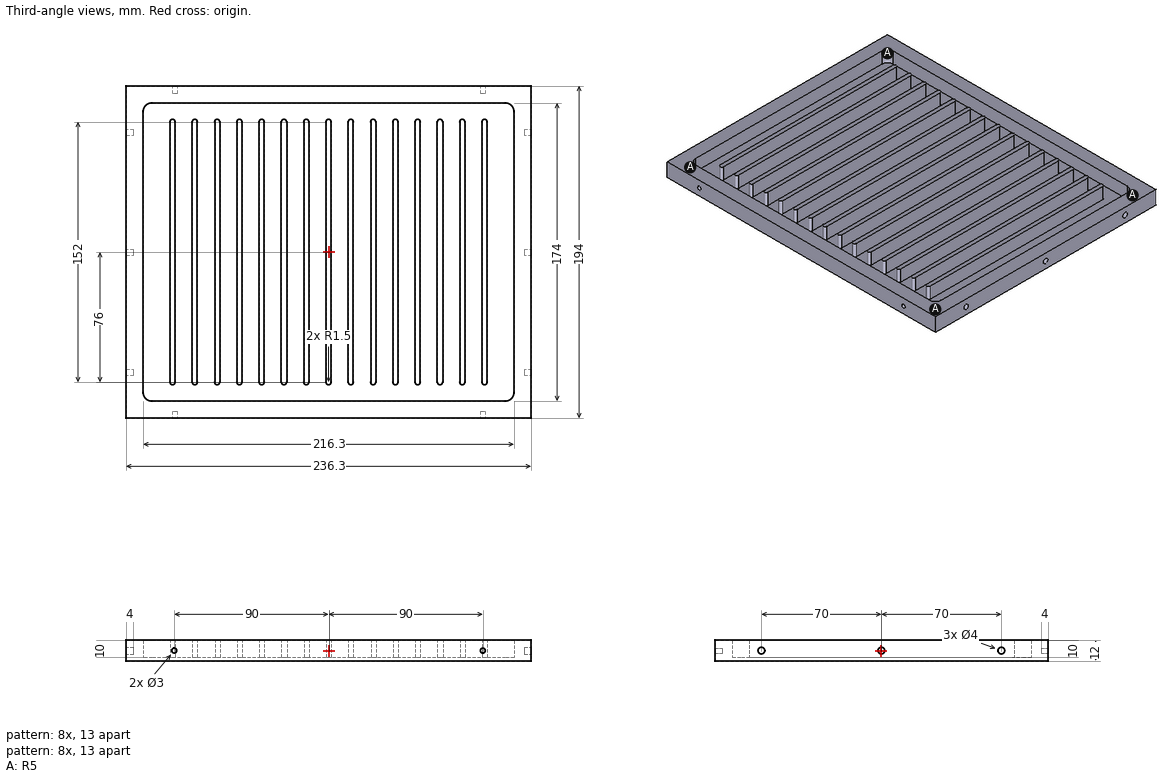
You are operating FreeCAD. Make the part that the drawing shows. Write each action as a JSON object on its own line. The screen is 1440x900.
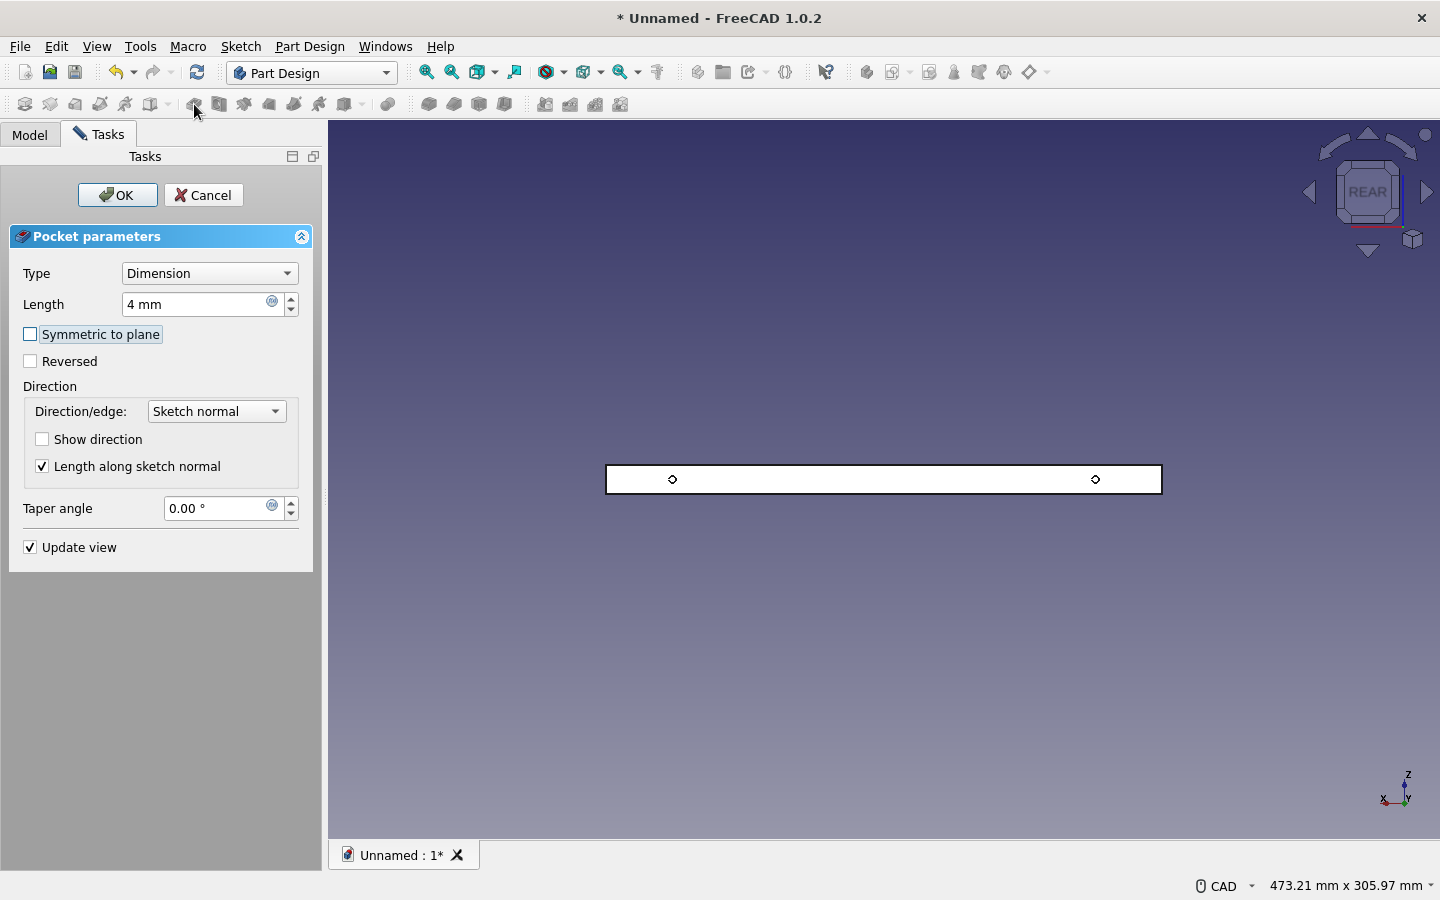
{"action": "left_click", "coordinate": [118, 195]}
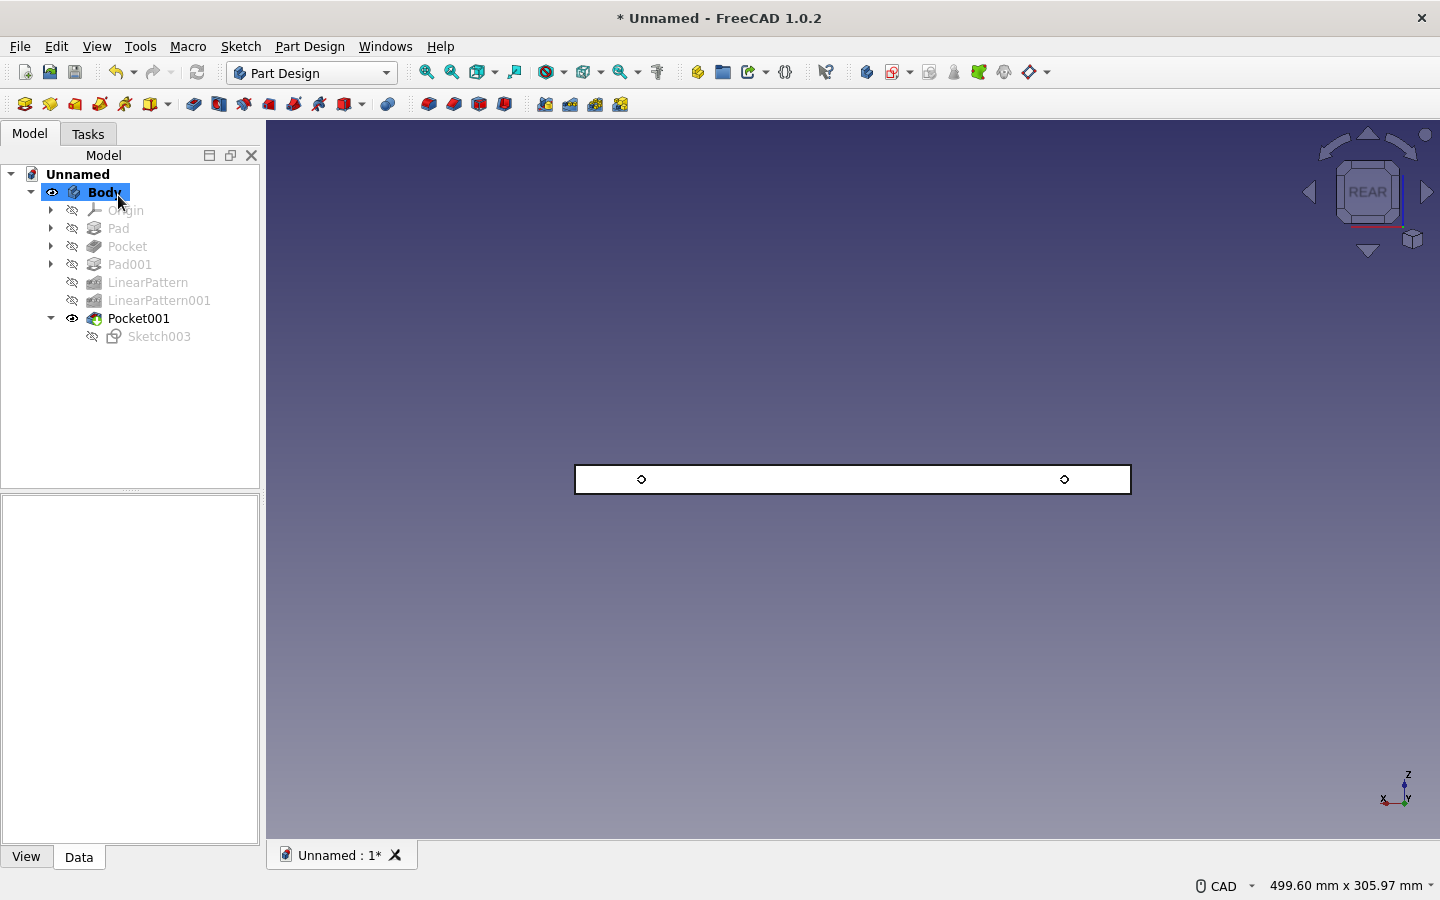
{"action": "left_click", "coordinate": [117, 318]}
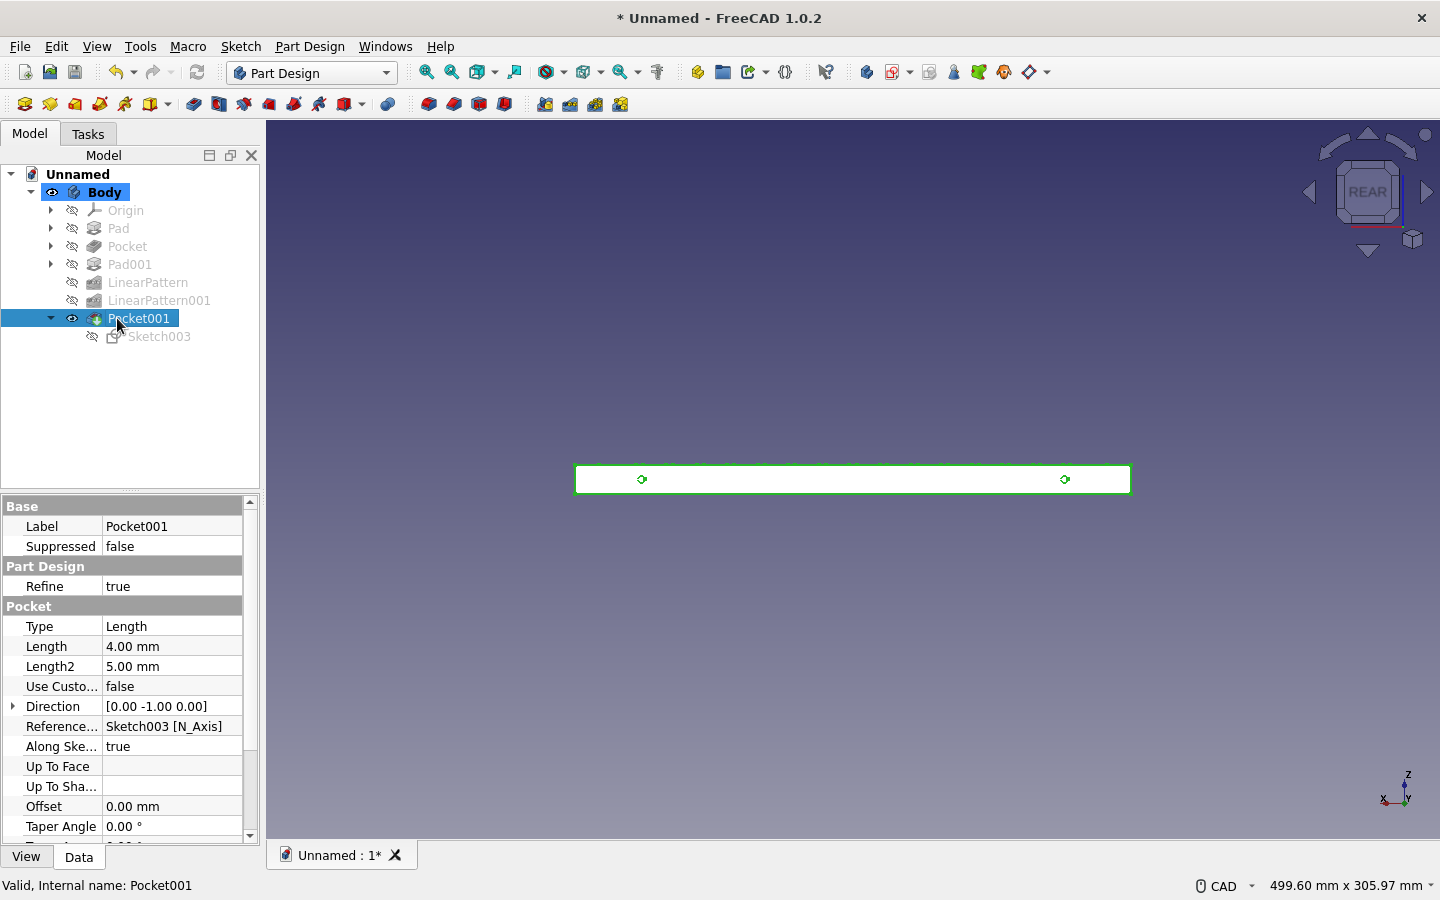
{"action": "left_click", "coordinate": [545, 104]}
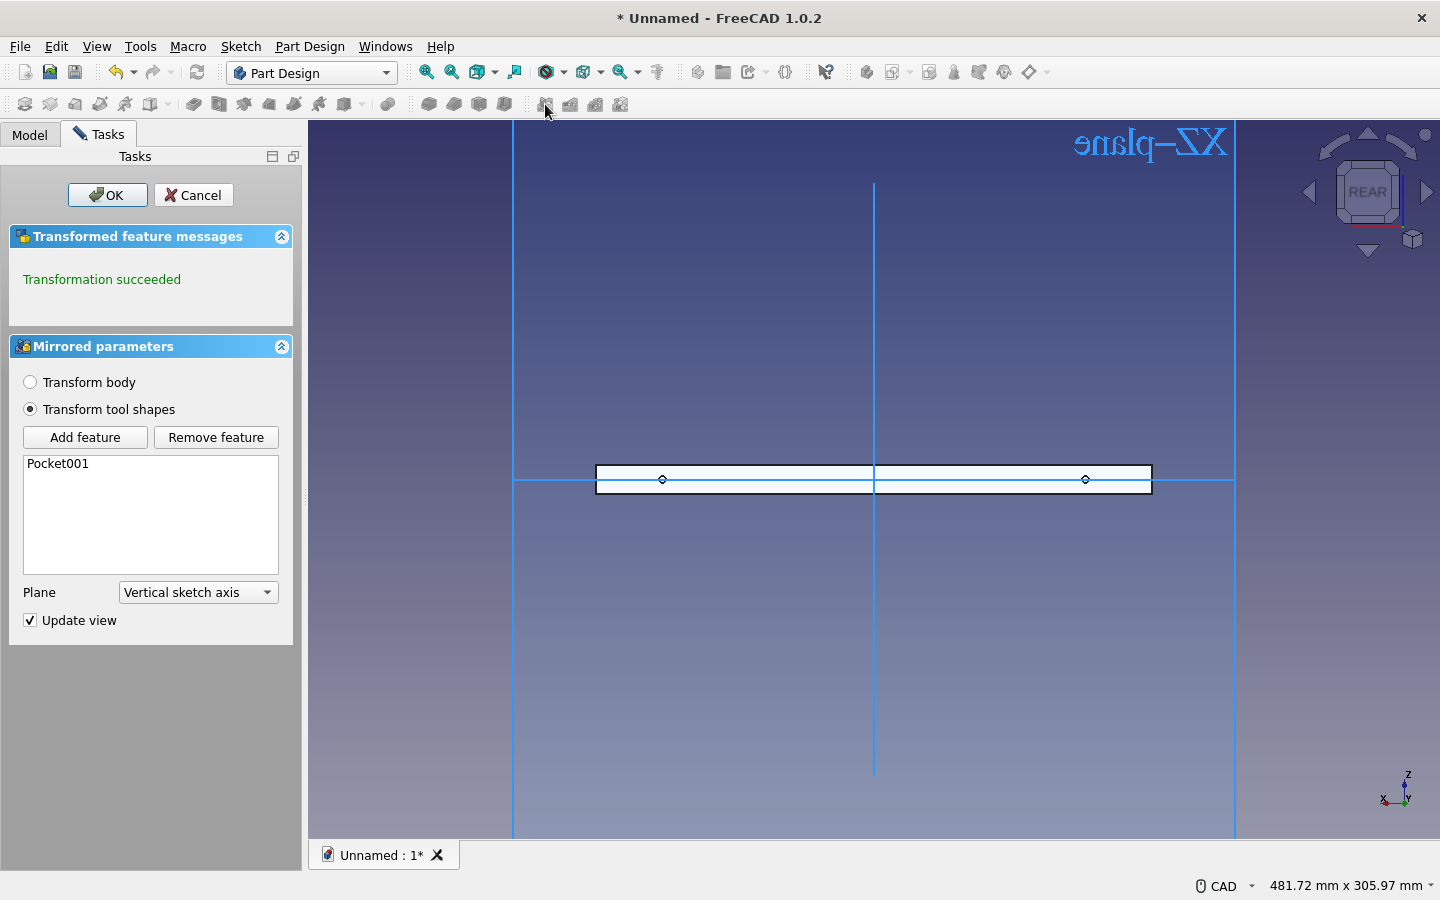
{"action": "left_click", "coordinate": [199, 592]}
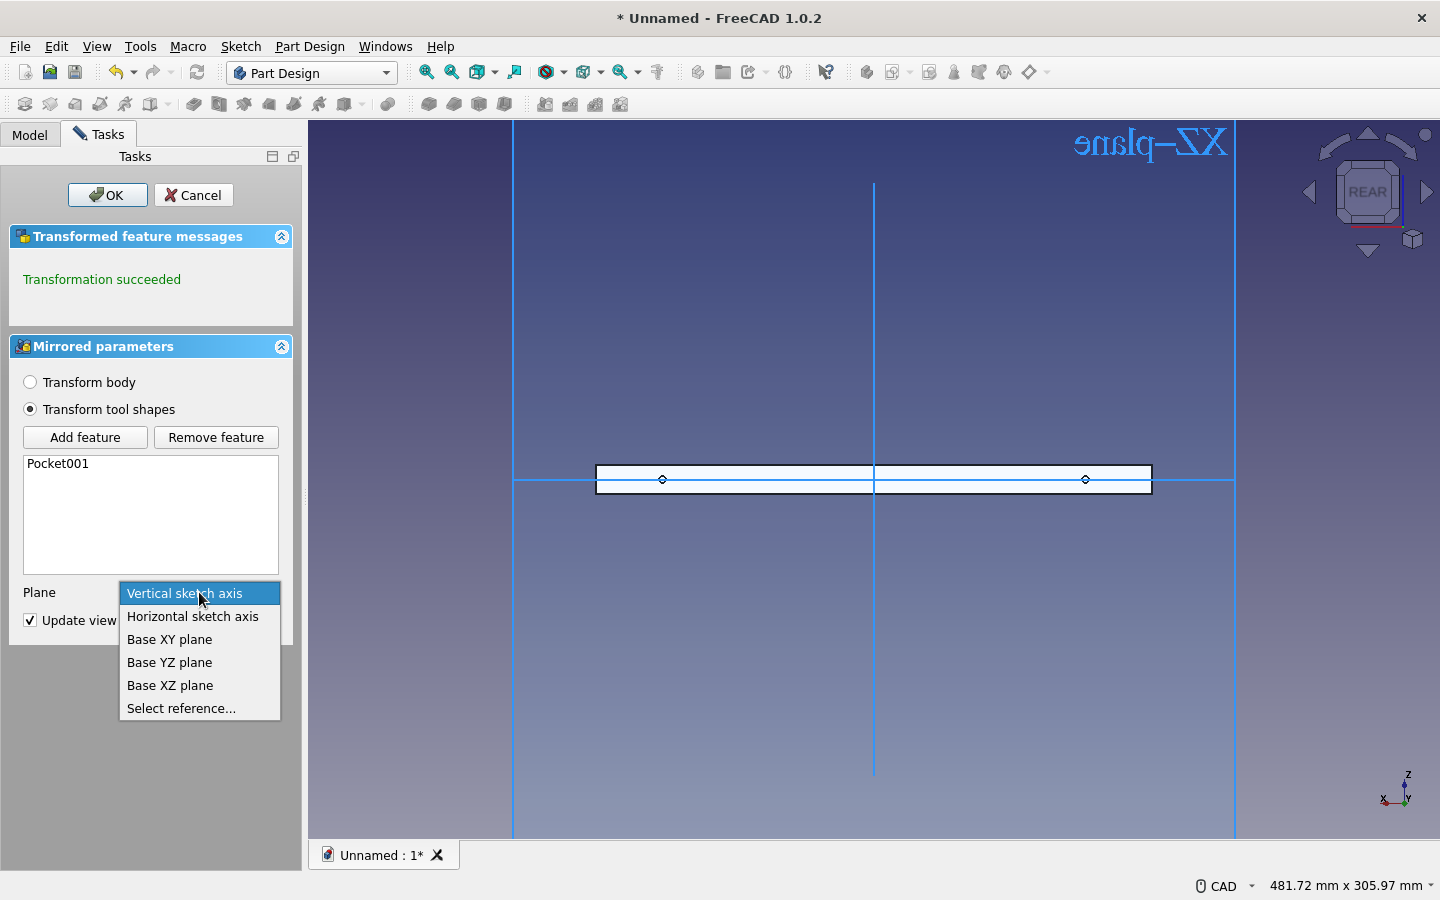
{"action": "left_click", "coordinate": [198, 686]}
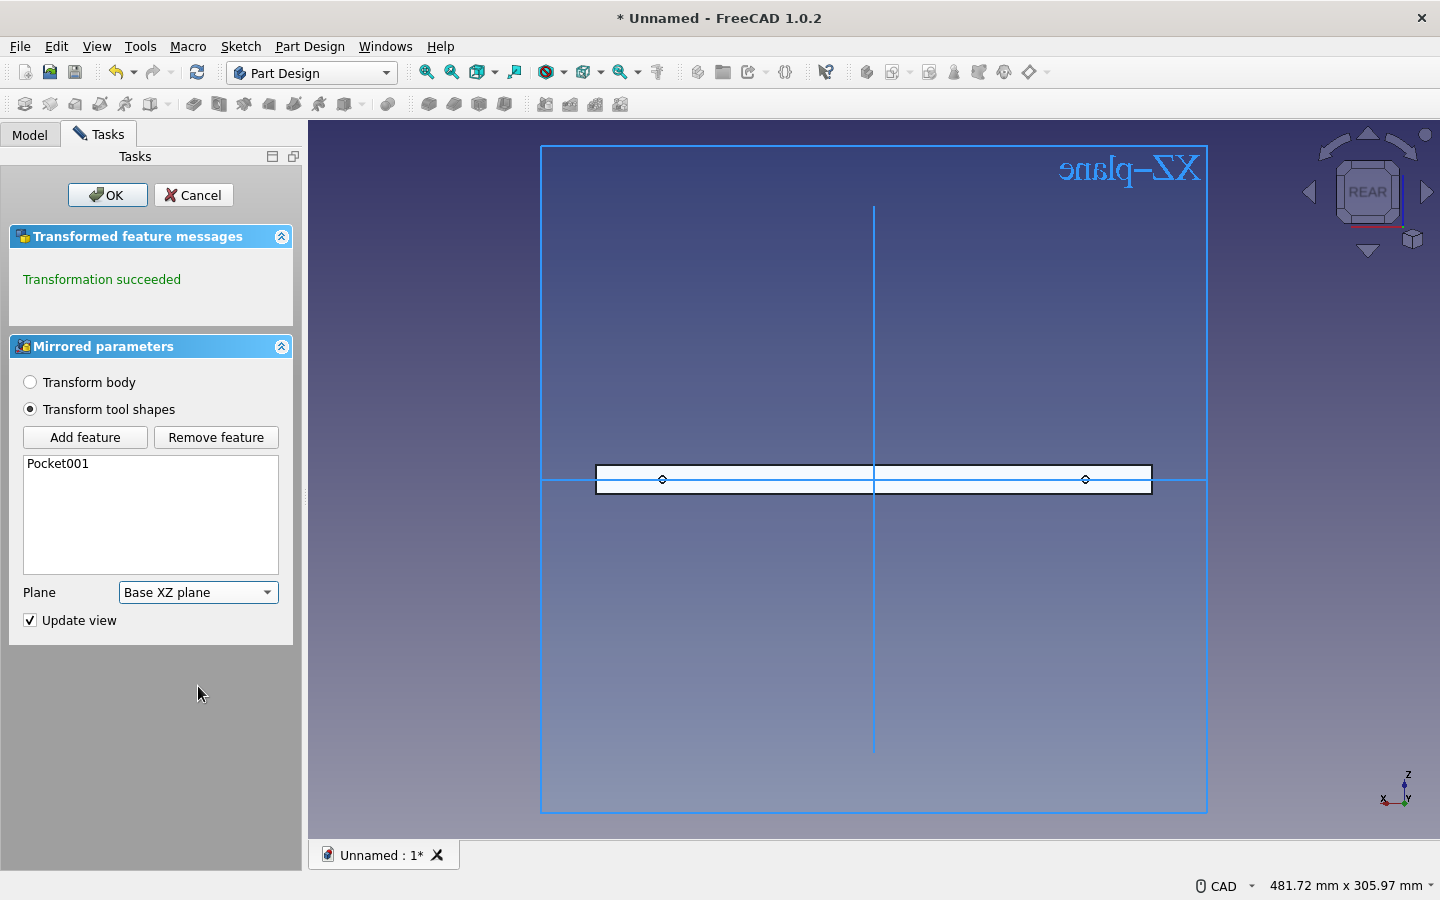
{"action": "left_click", "coordinate": [108, 195]}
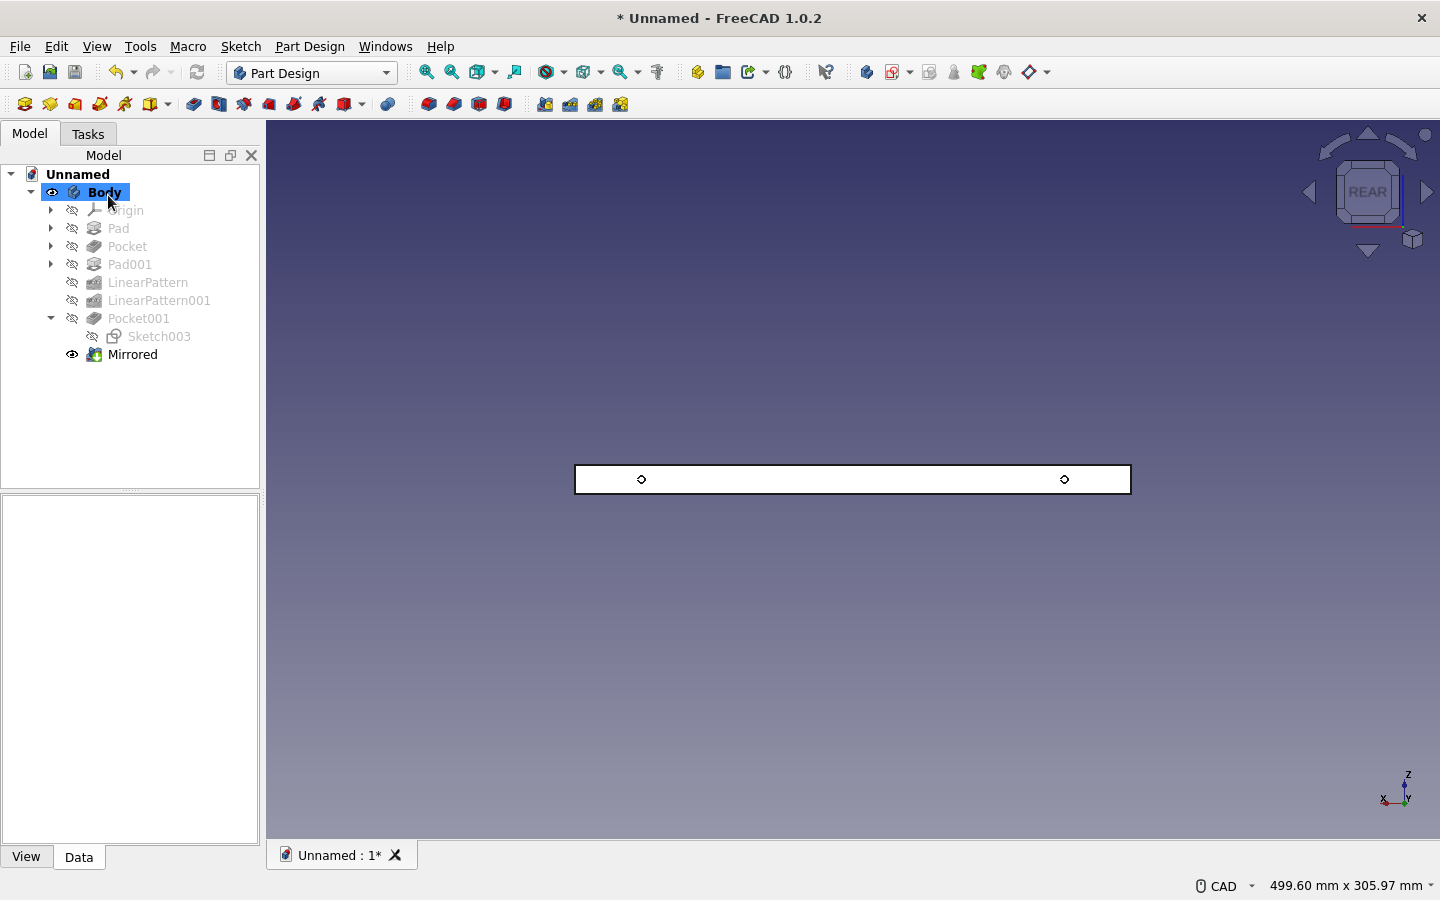
{"action": "key", "text": "6"}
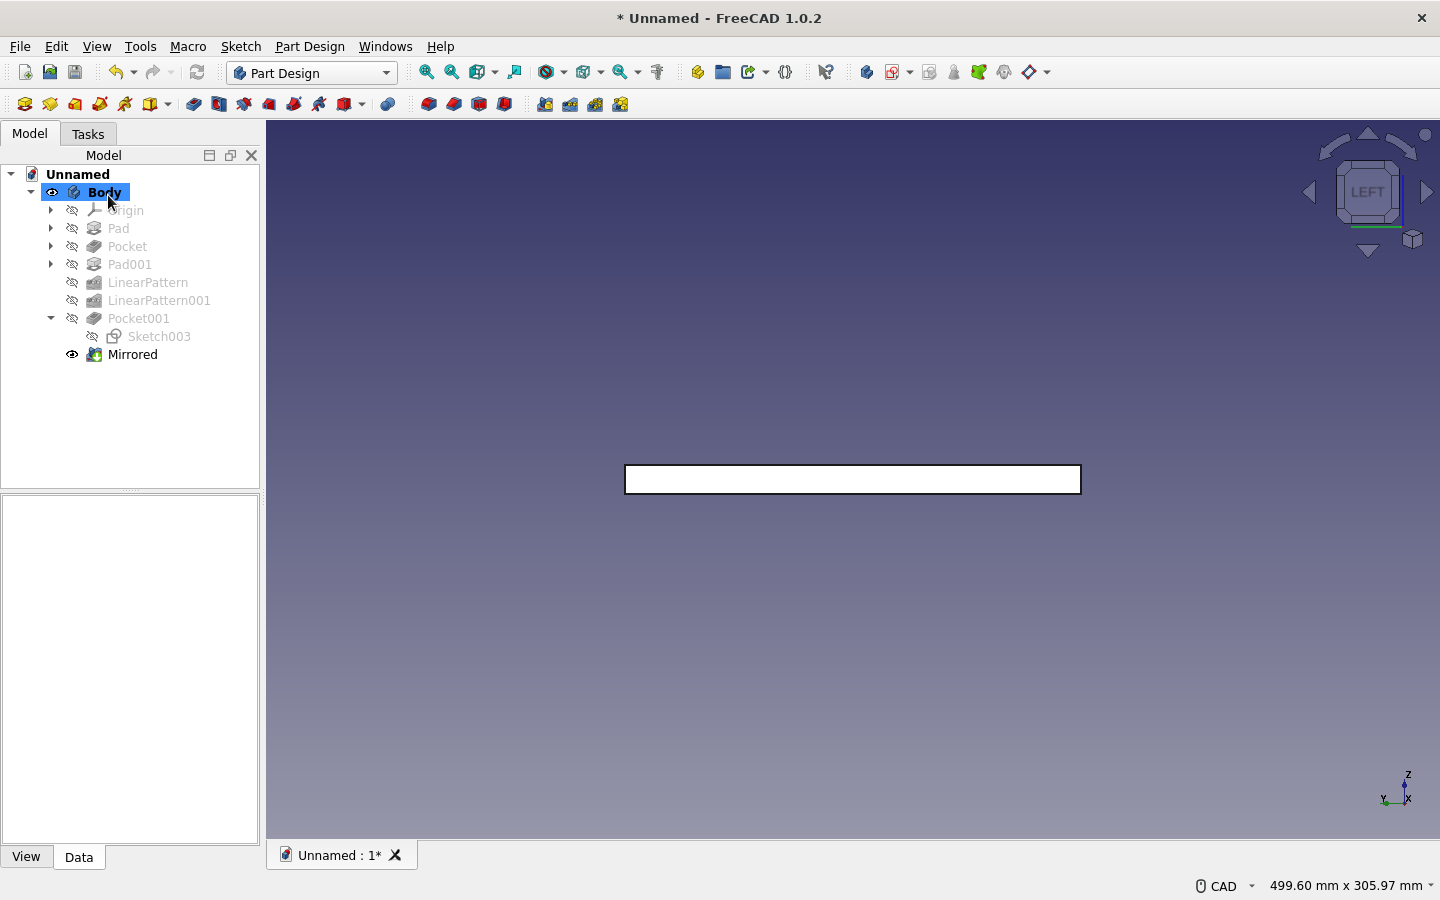
{"action": "left_click", "coordinate": [427, 72]}